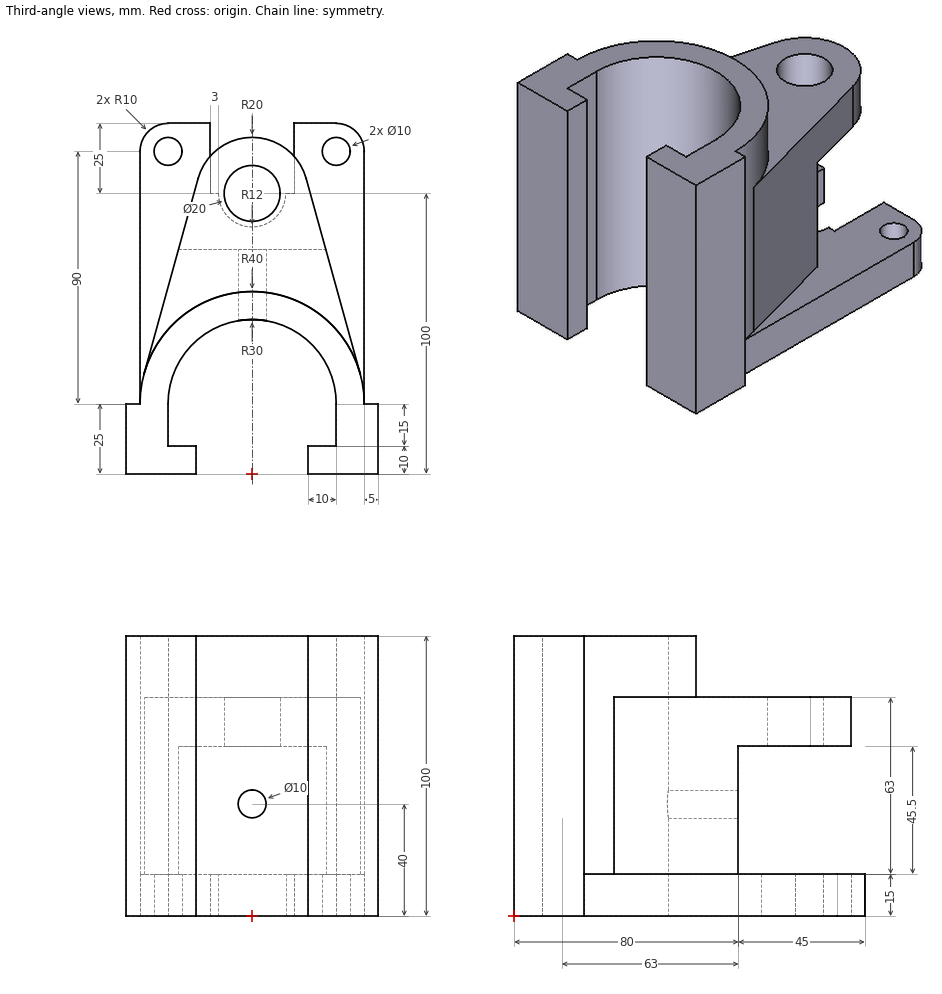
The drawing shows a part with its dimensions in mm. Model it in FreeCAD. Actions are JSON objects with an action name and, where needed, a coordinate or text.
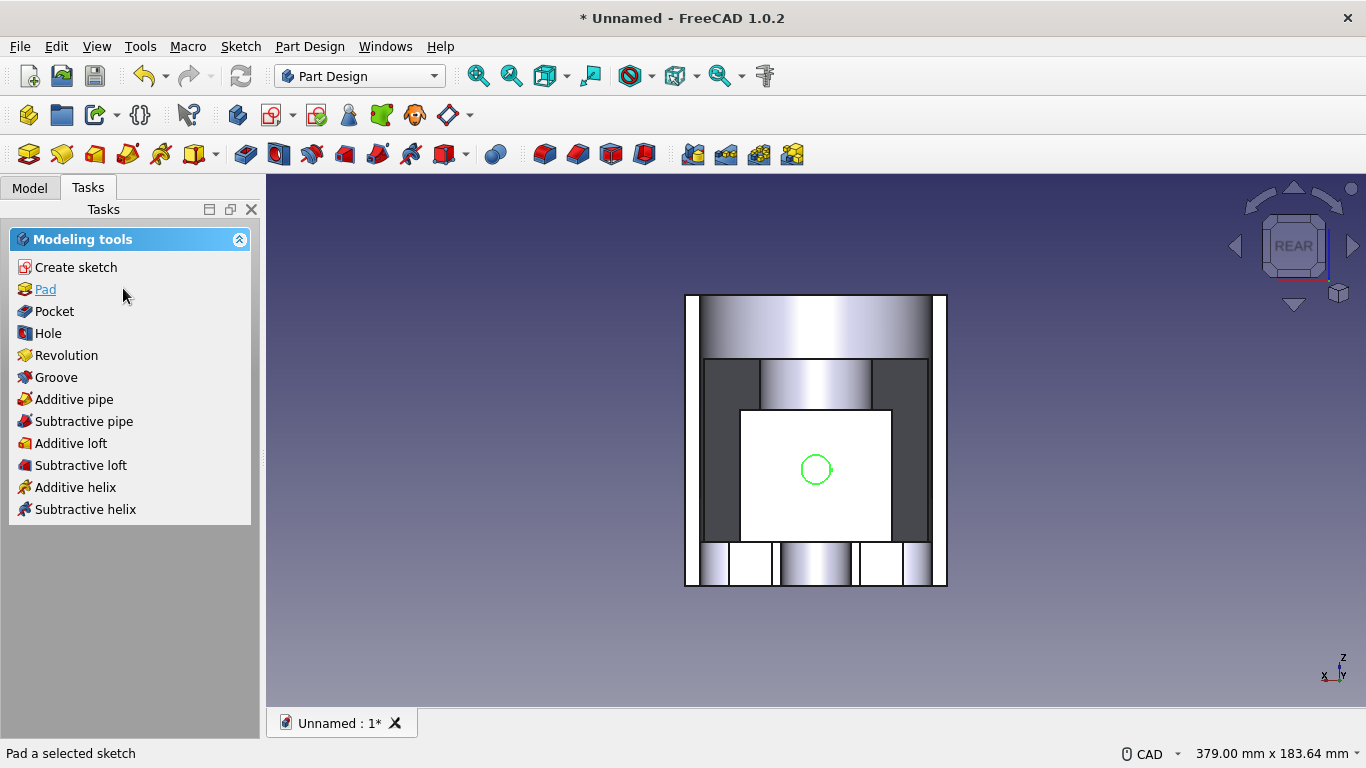
{"action": "left_click", "coordinate": [246, 154]}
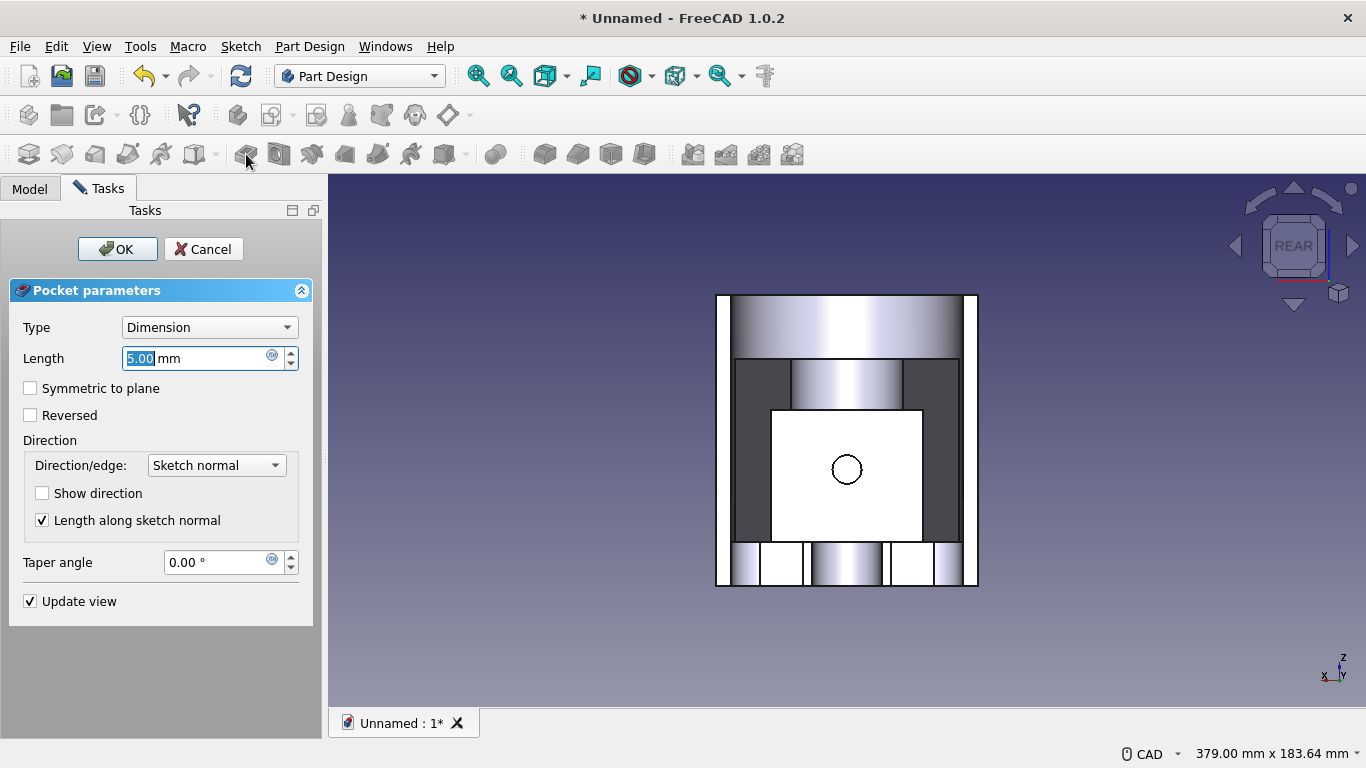
{"action": "type", "text": "63"}
{"action": "key", "text": "Tab"}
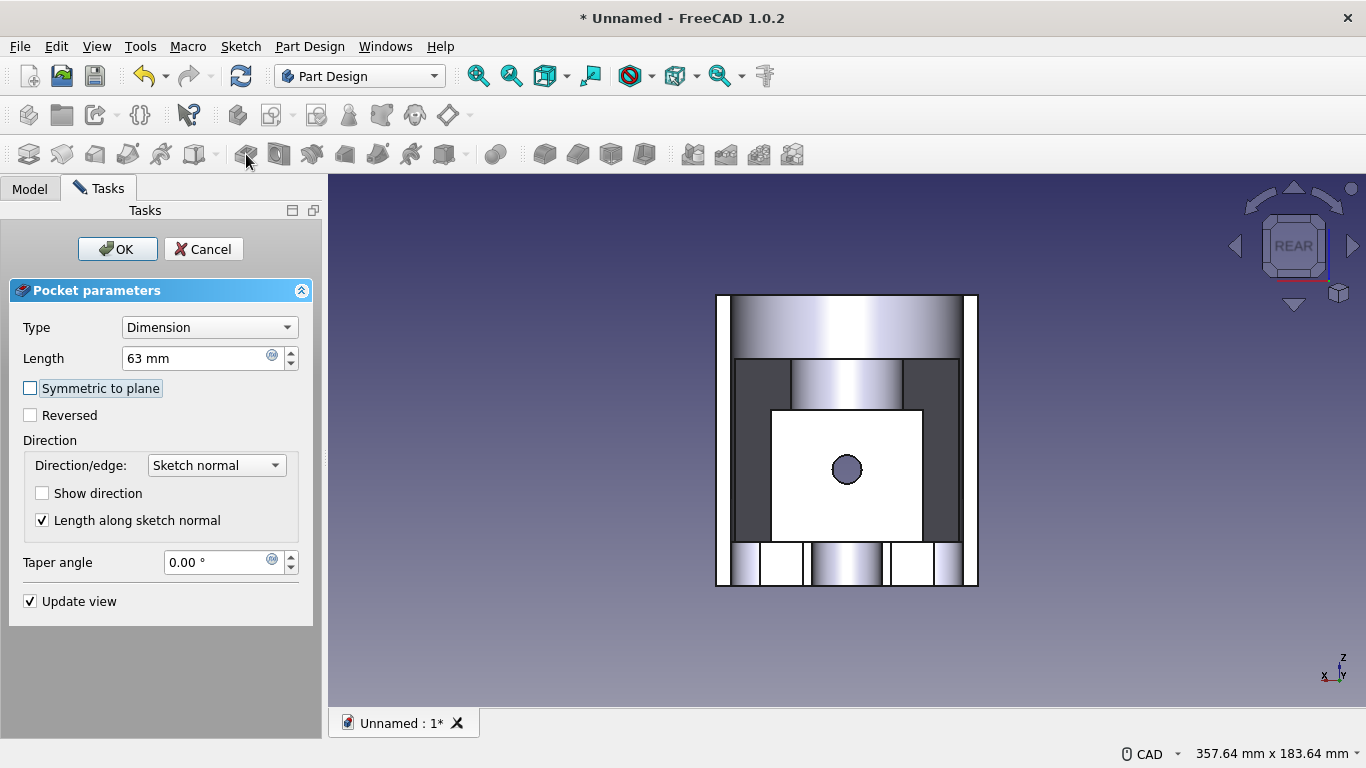
{"action": "left_click", "coordinate": [118, 249]}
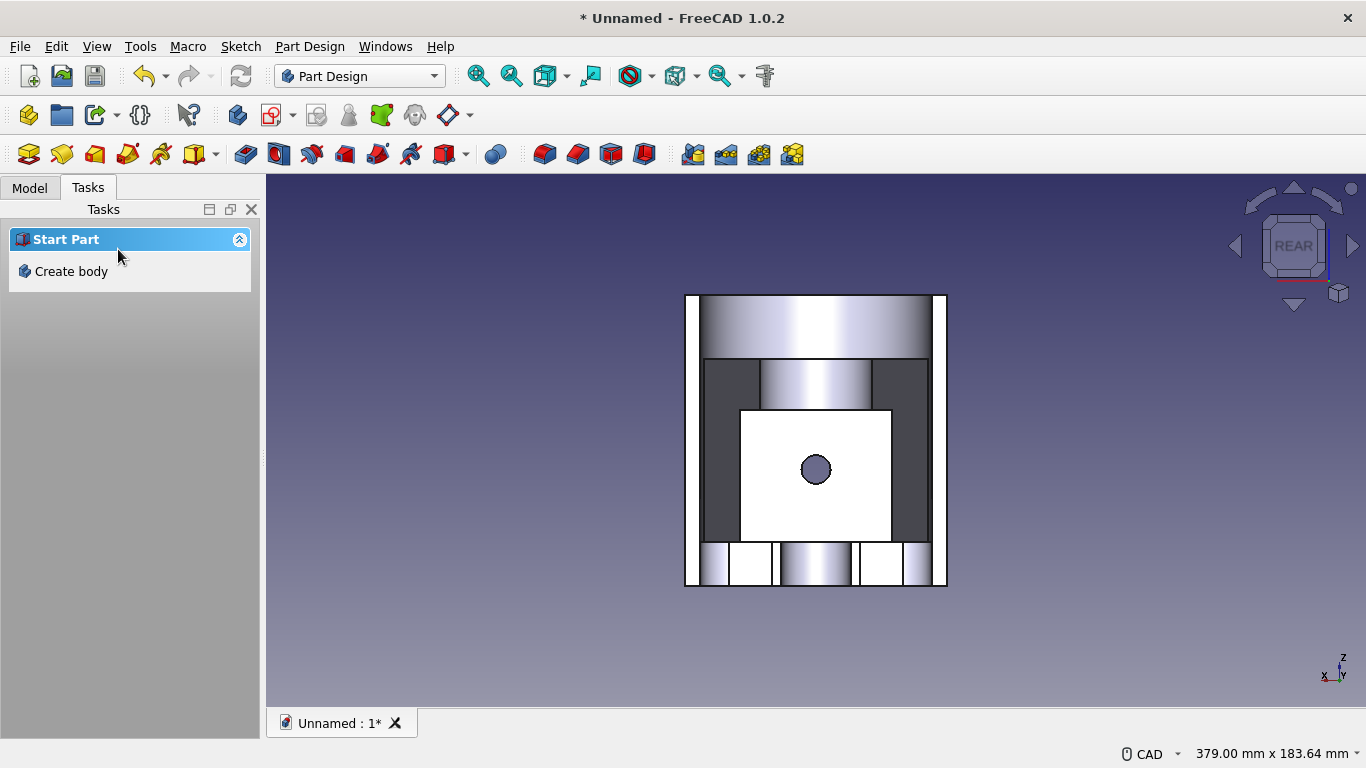
{"action": "key", "text": "0"}